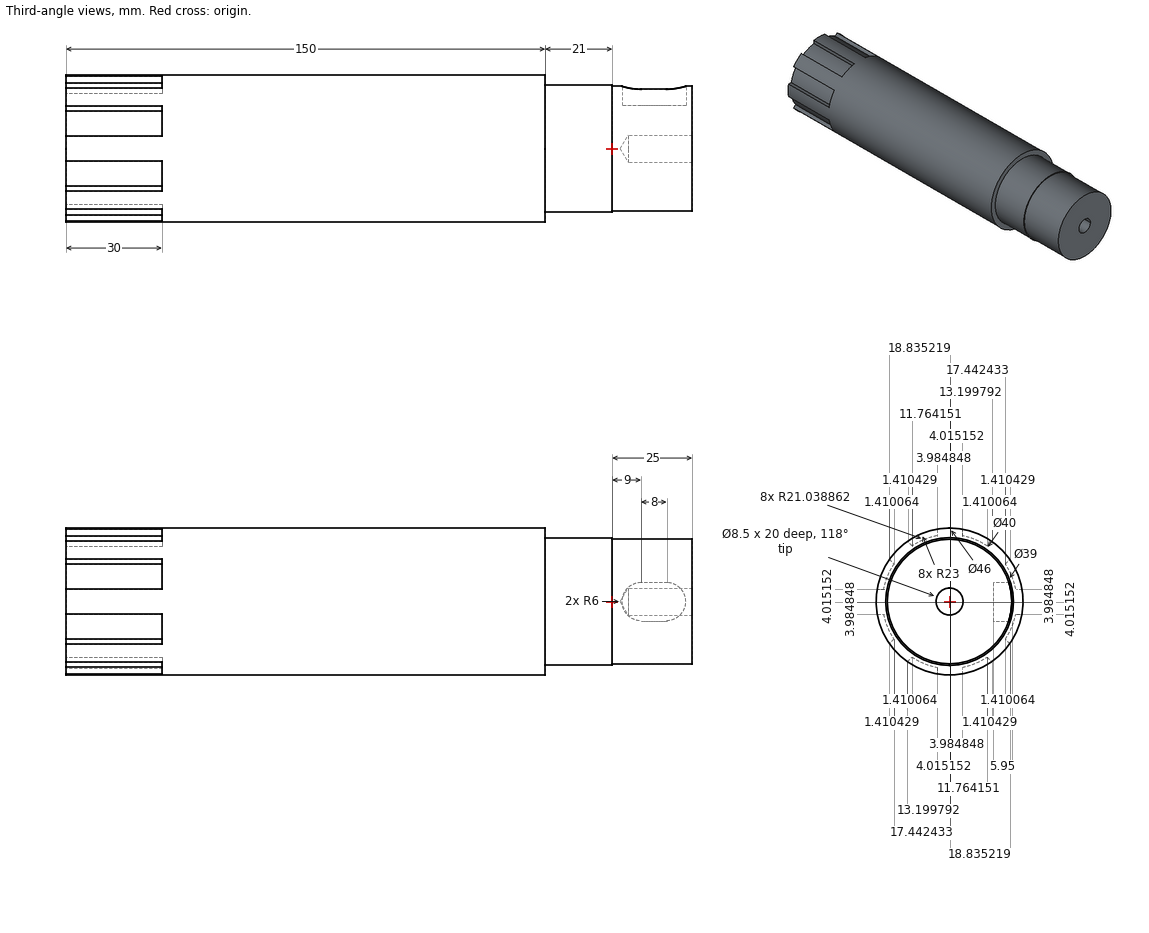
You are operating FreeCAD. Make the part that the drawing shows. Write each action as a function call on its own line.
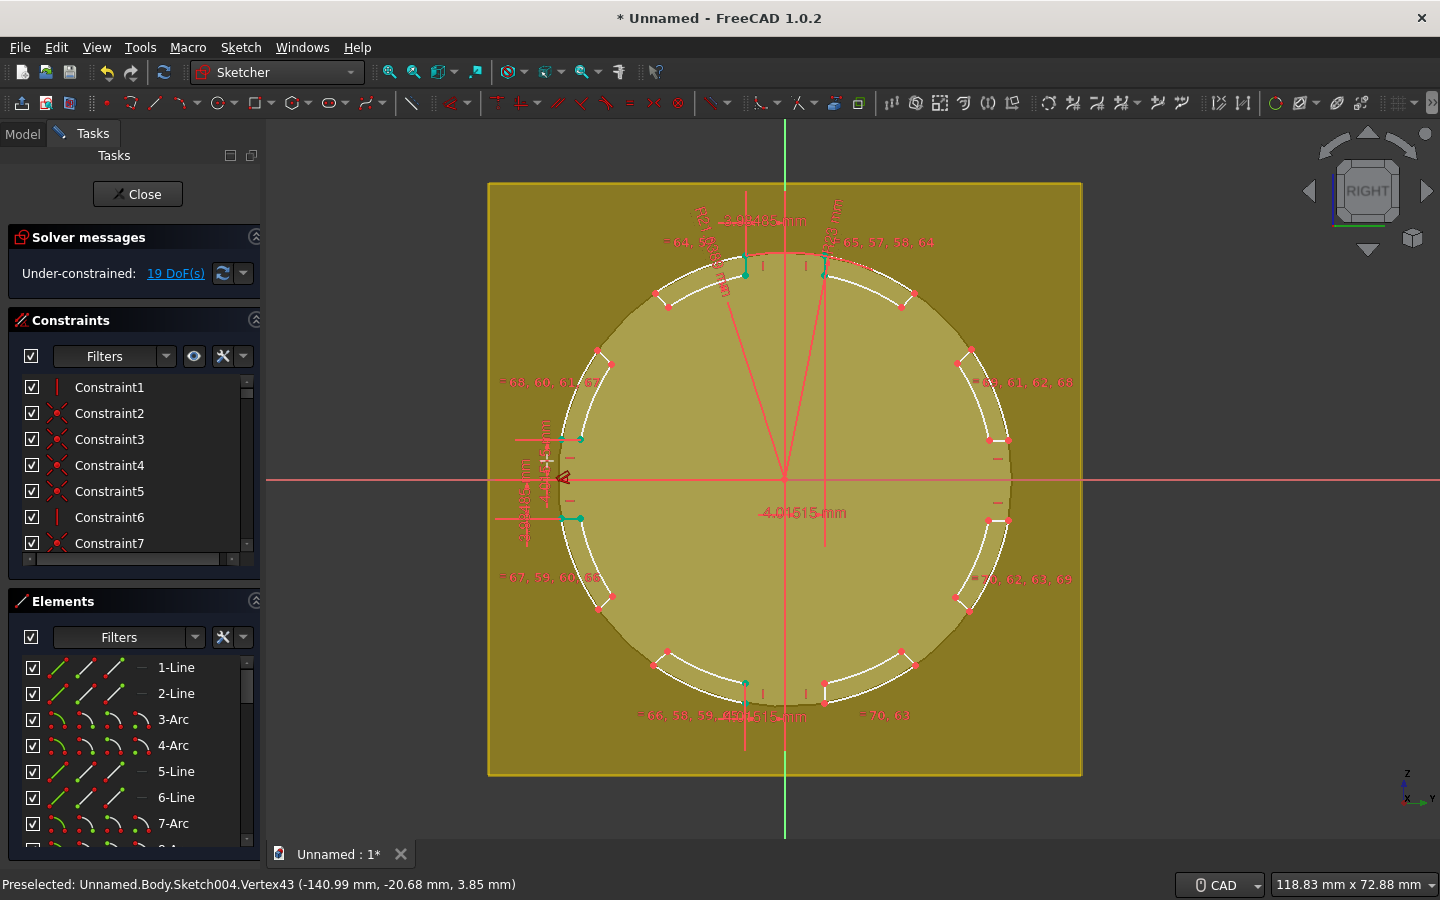
click(1009, 441)
click(1043, 460)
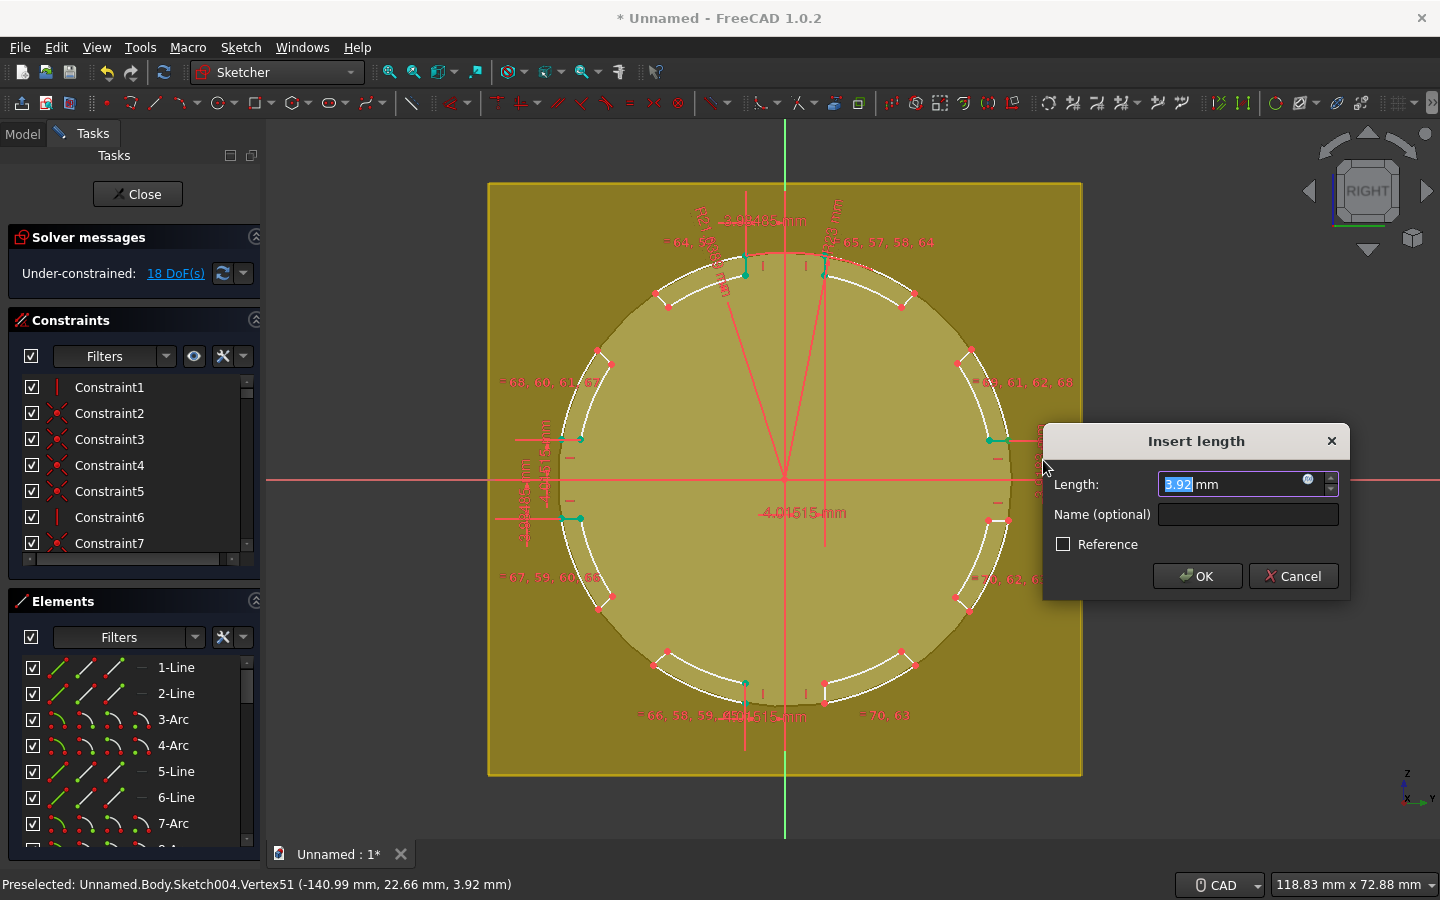
text(3.984848)
key(Return)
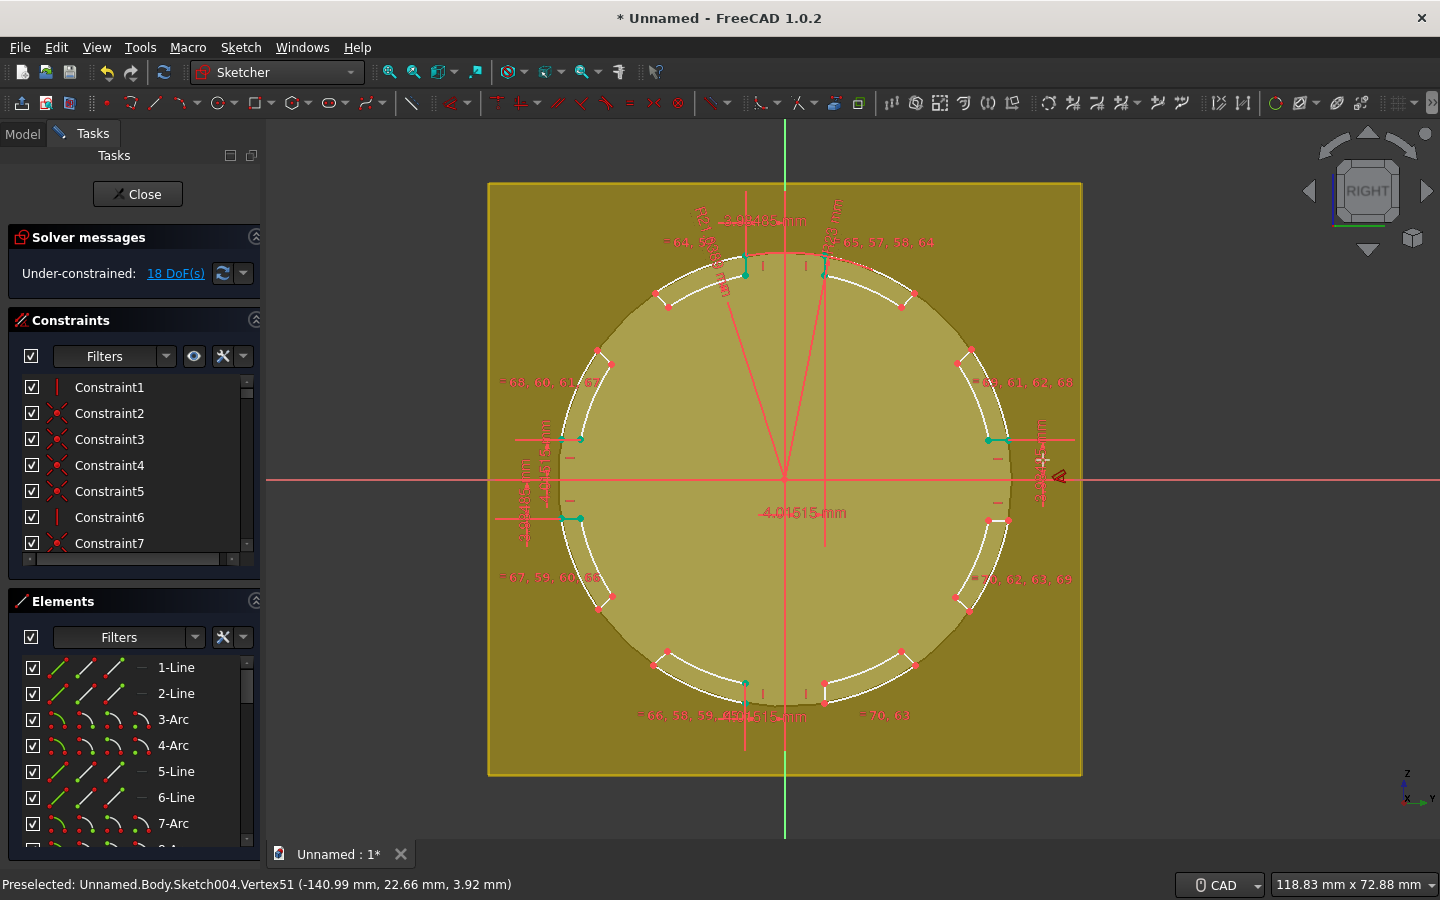
click(989, 521)
click(1023, 500)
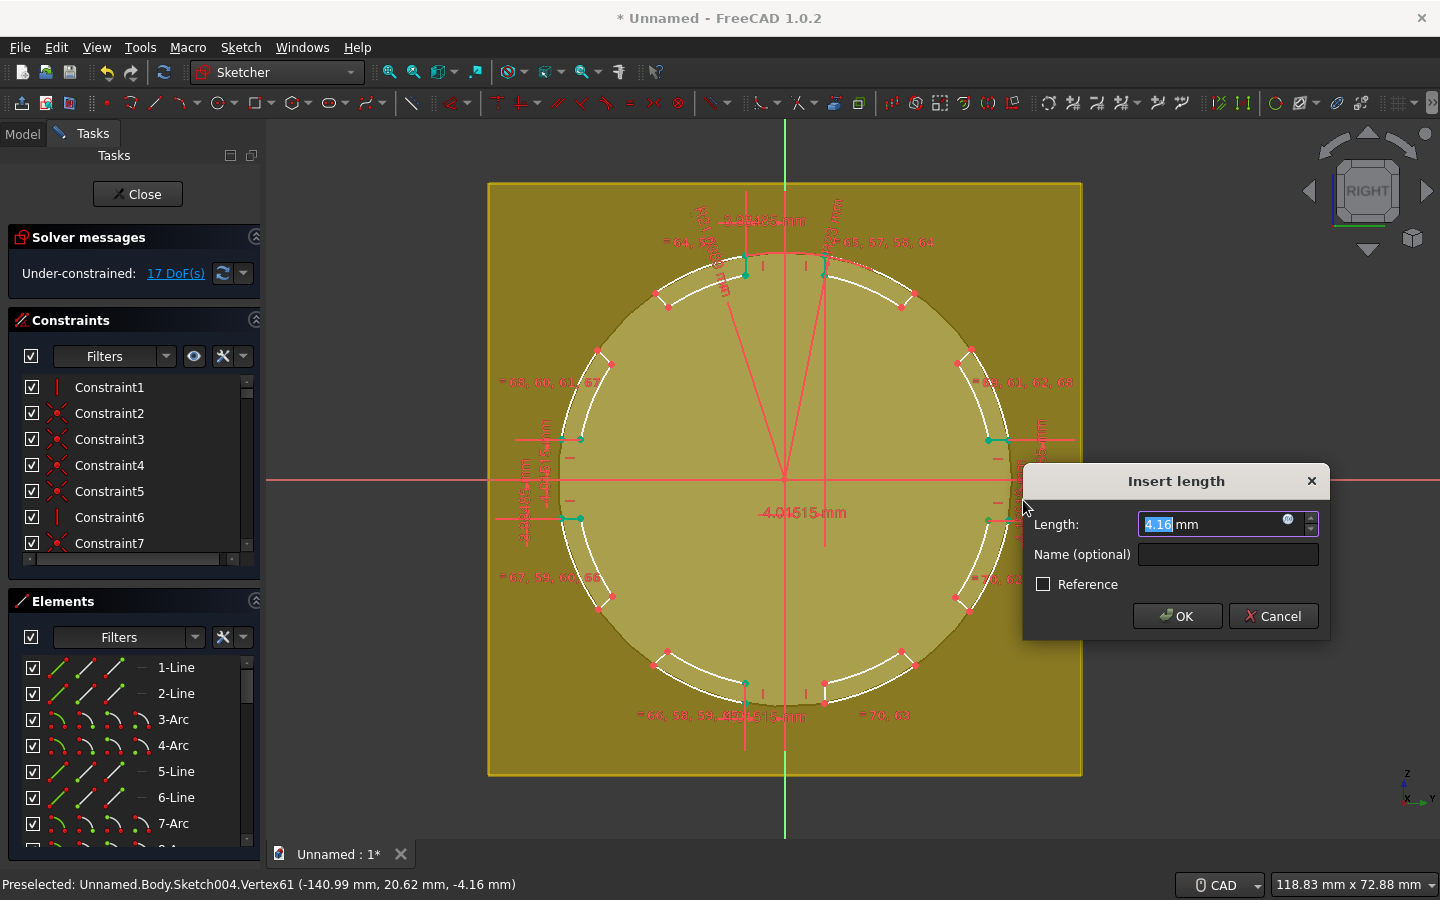
text(4.015152)
key(Return)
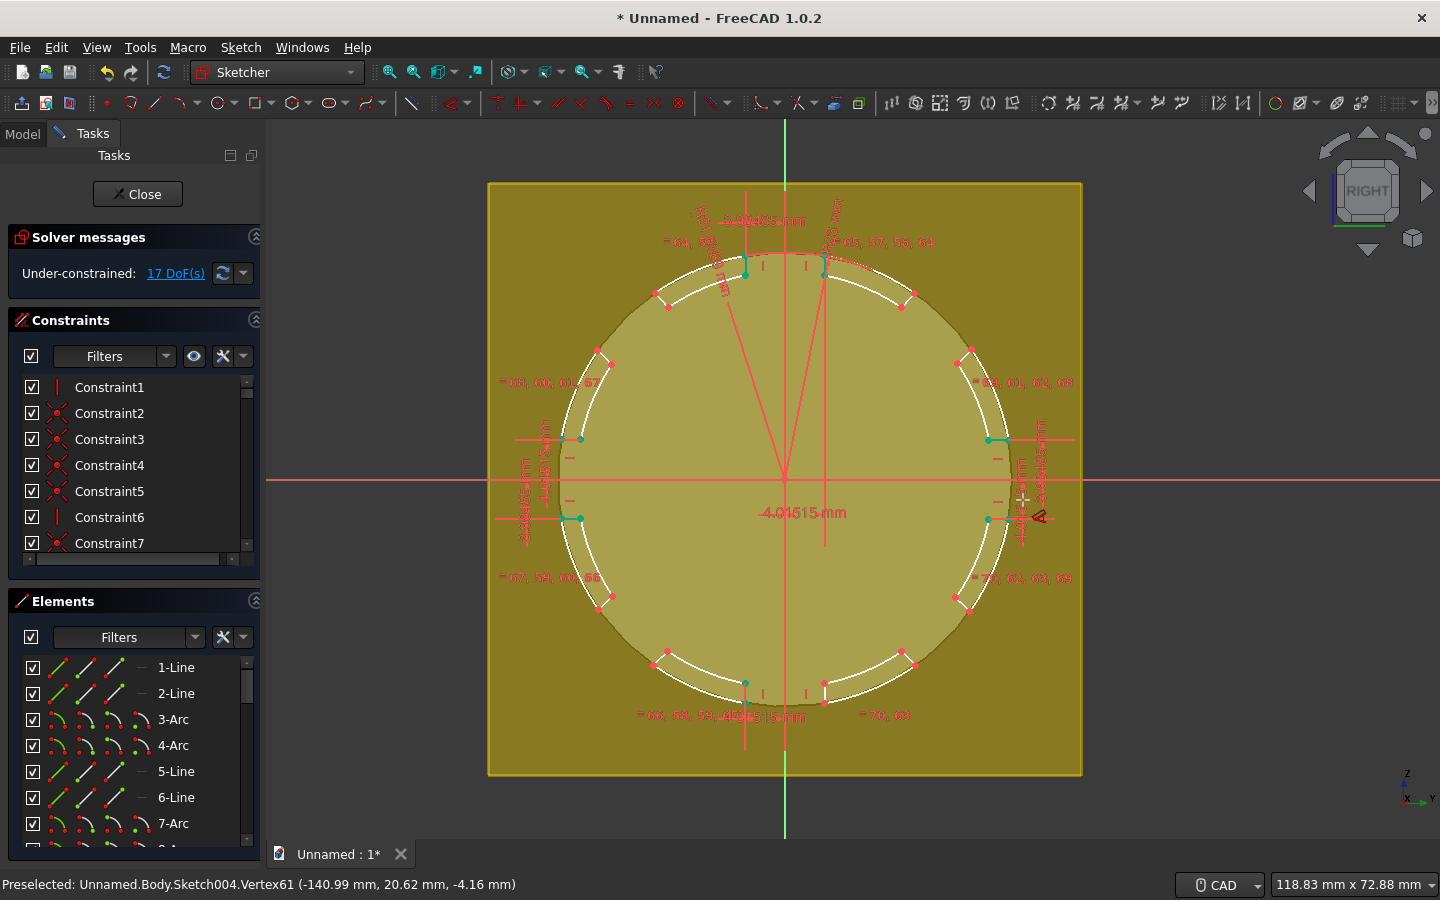
click(825, 703)
click(805, 446)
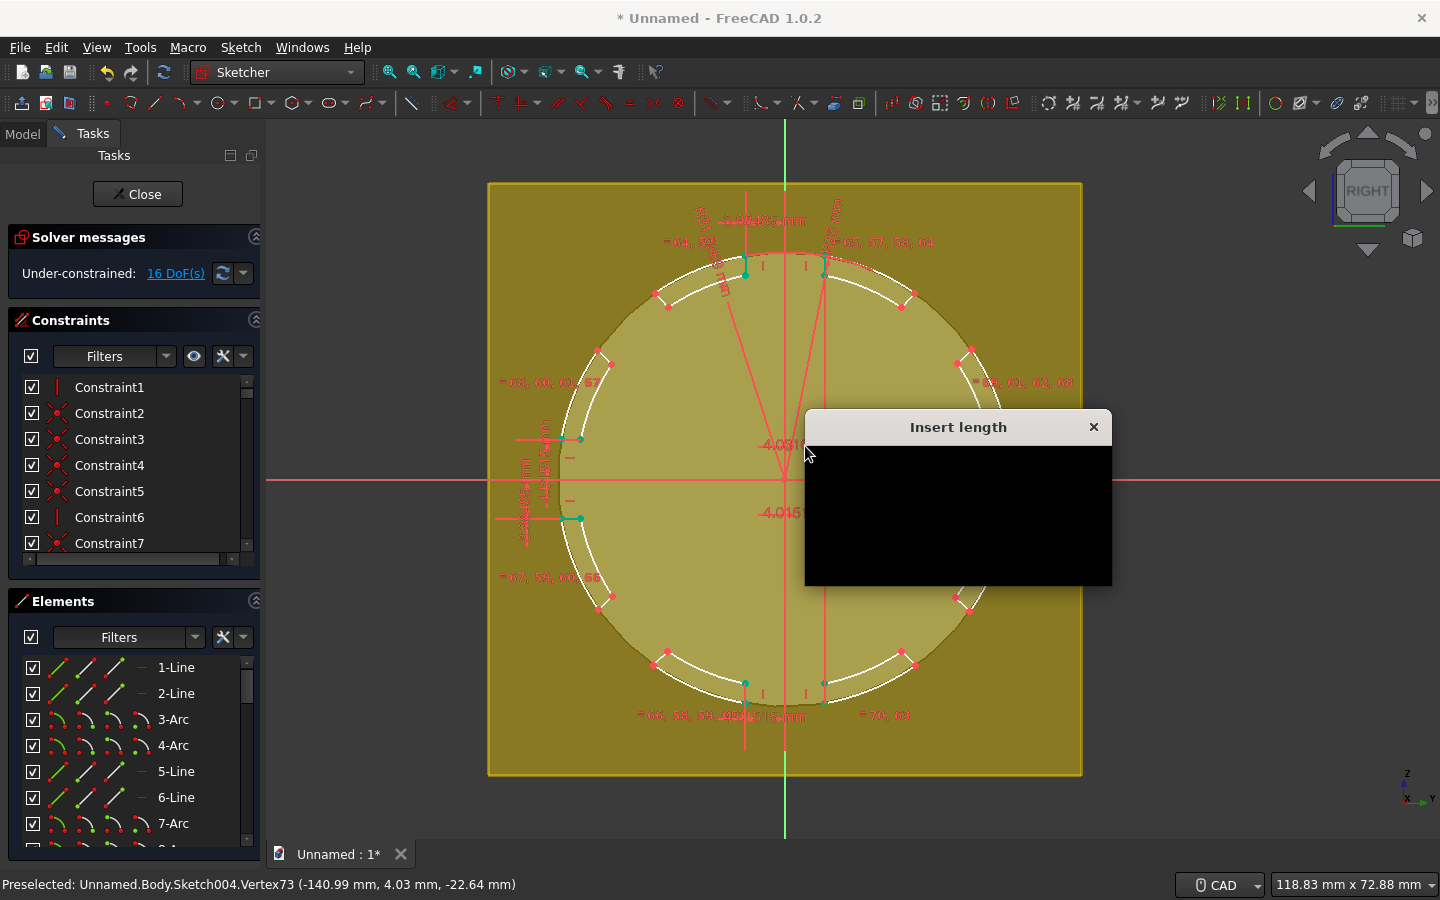
text(3.984848)
key(Return)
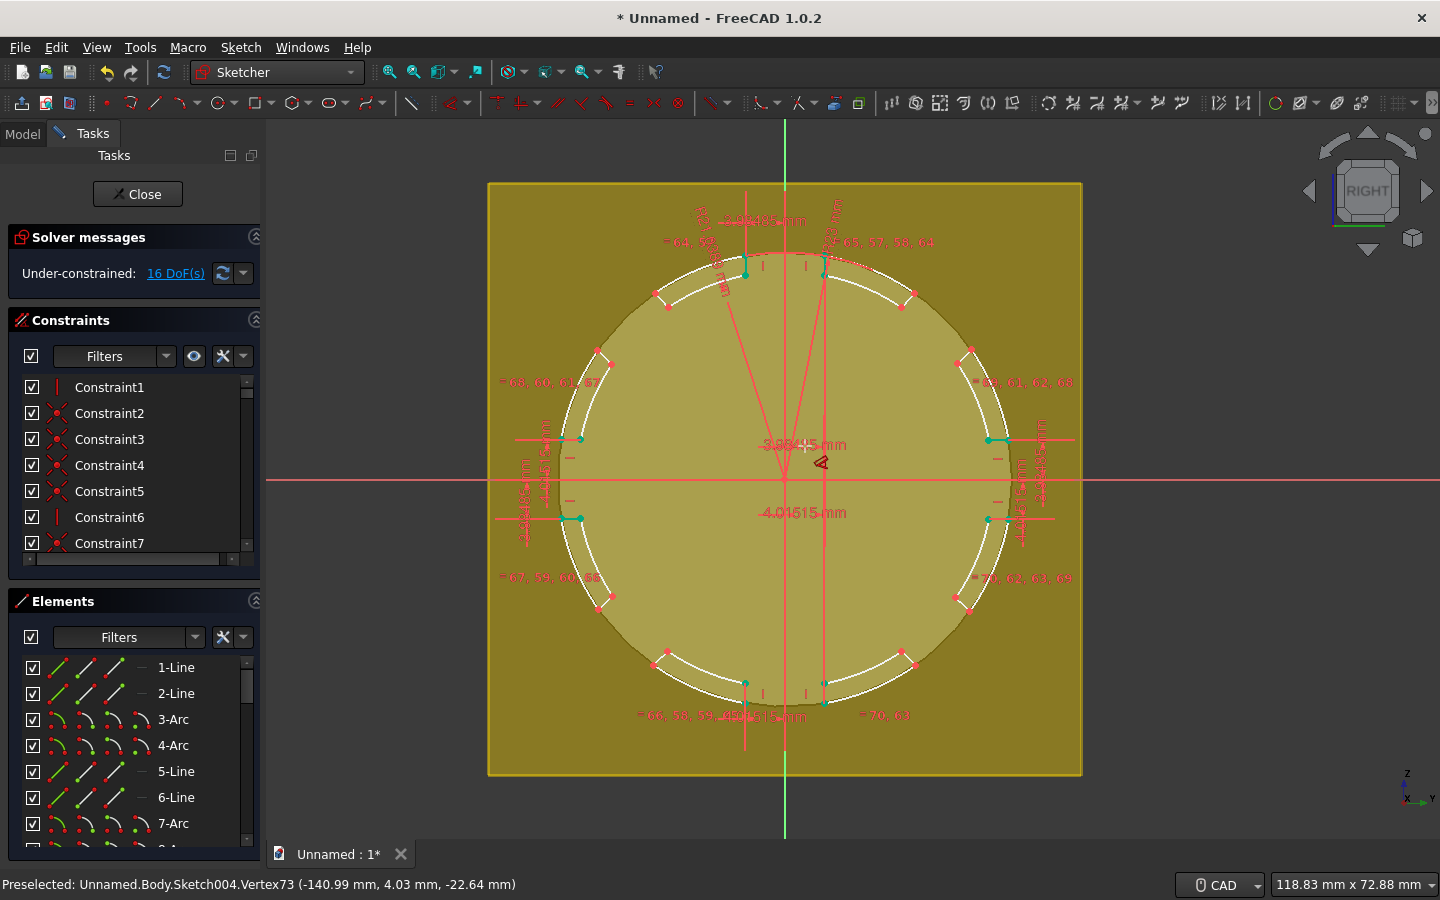
scroll(662, 300, up, 6)